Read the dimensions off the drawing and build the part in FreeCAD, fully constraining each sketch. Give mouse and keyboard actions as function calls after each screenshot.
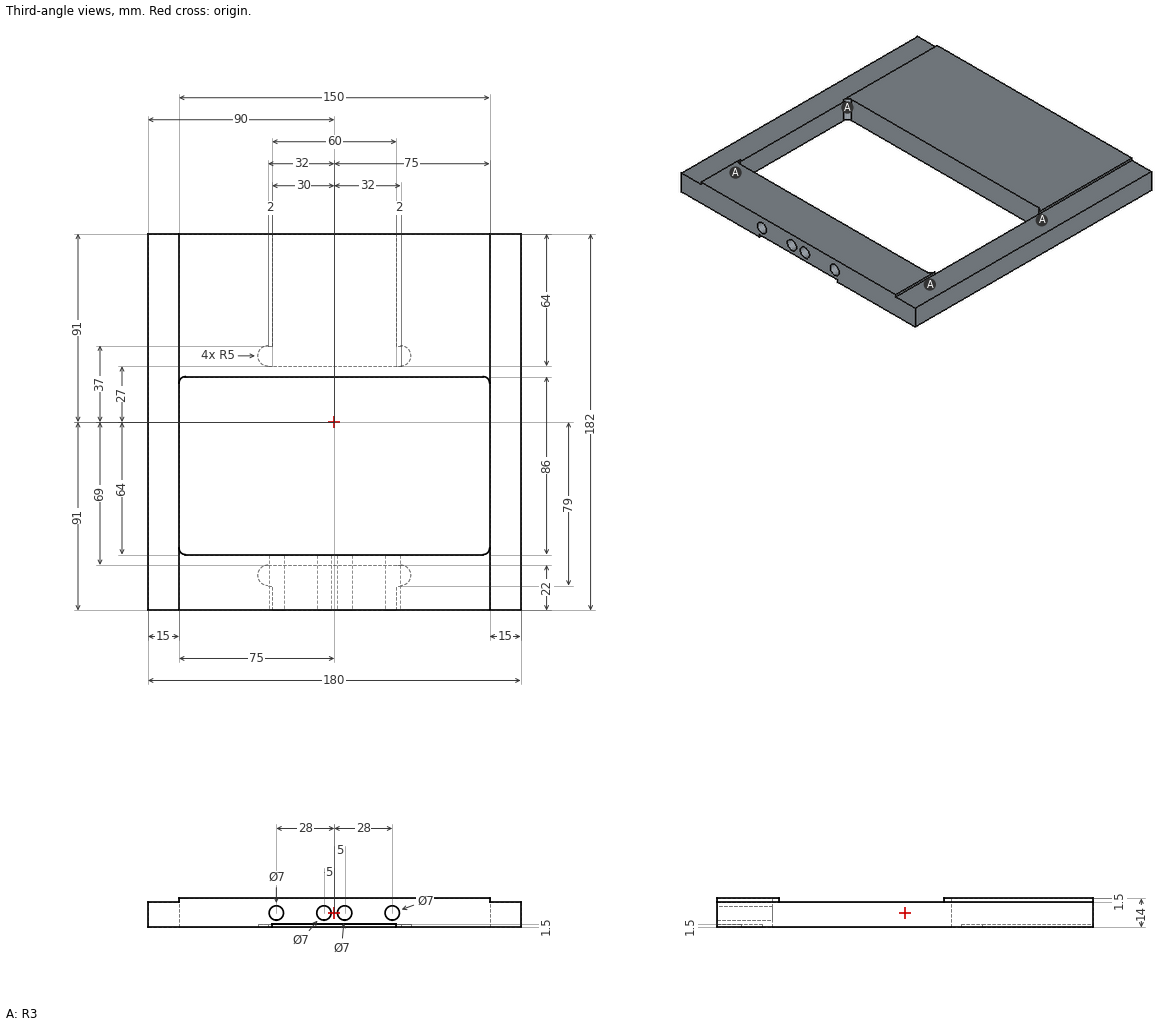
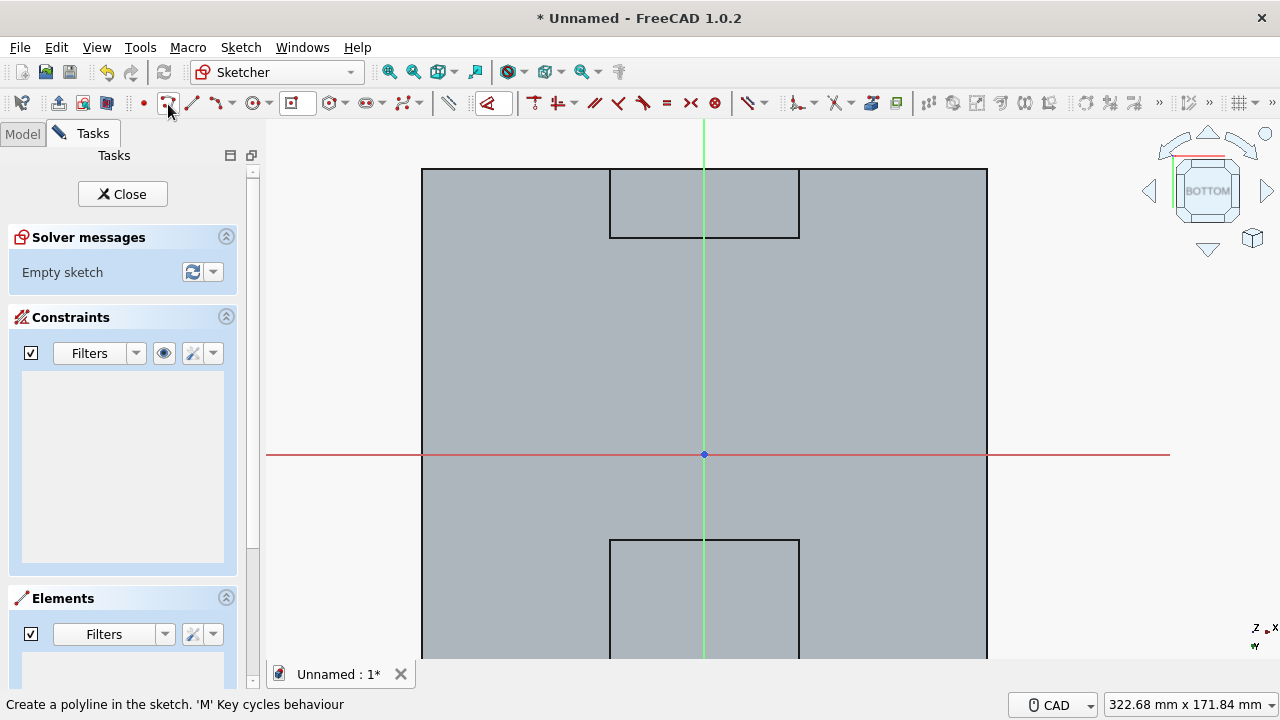
click(604, 571)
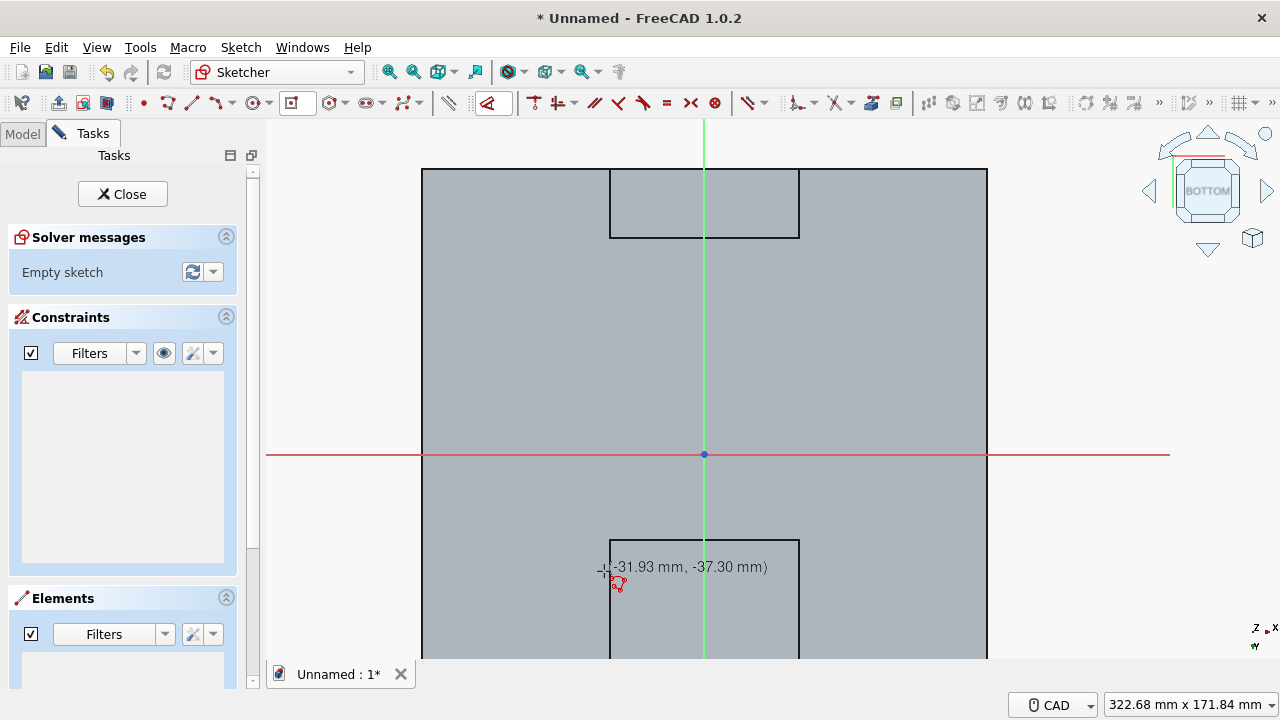
scroll(610, 571, up, 5)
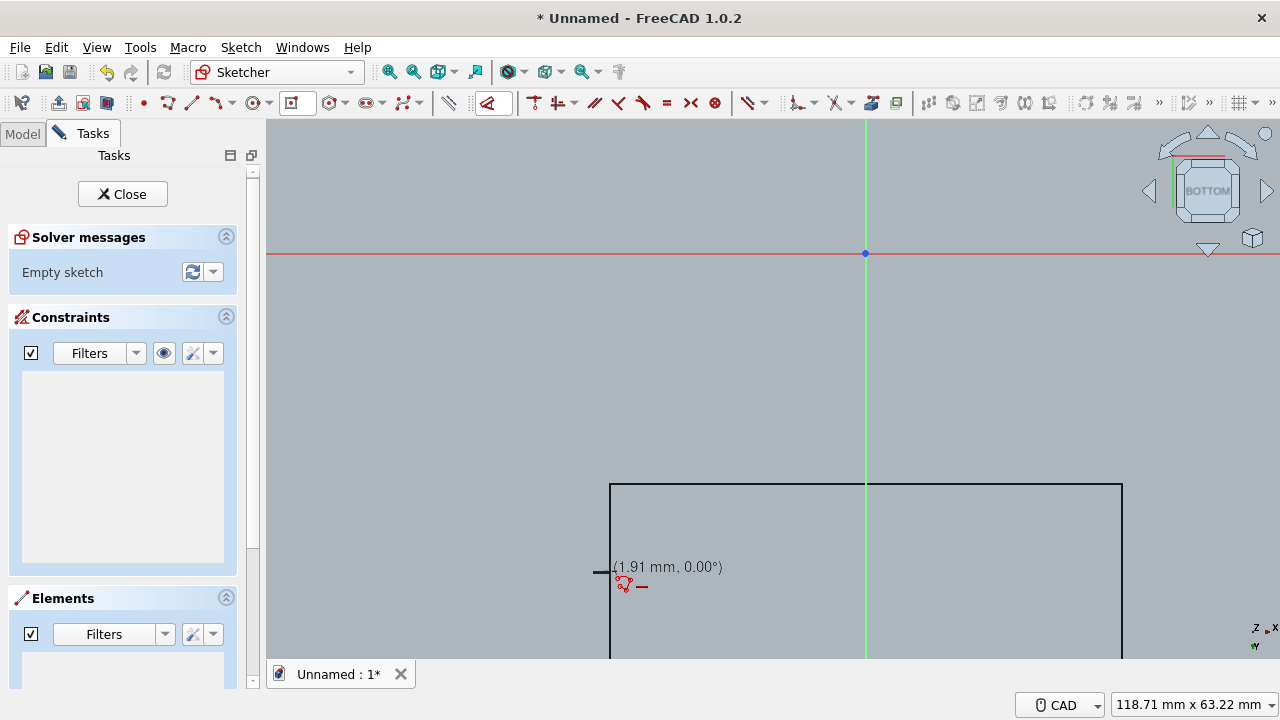
click(610, 570)
click(610, 484)
click(592, 484)
right_click(592, 484)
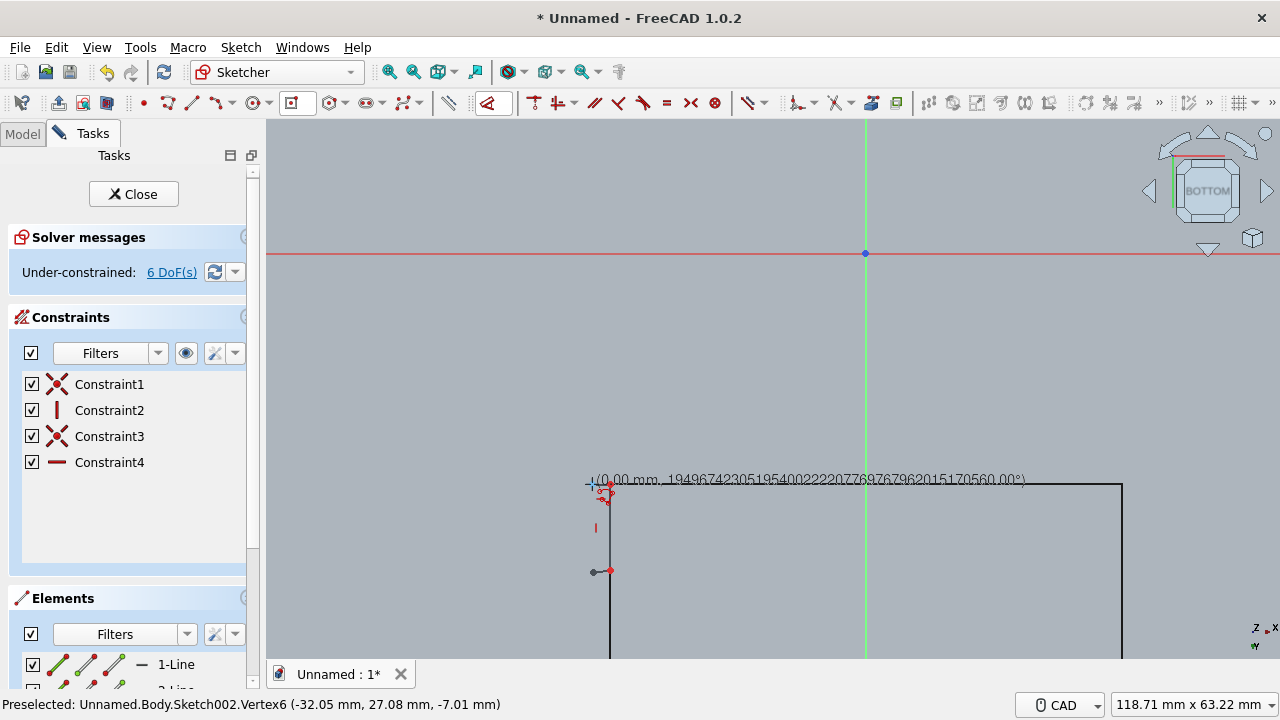
key(g)
key(3)
key(a)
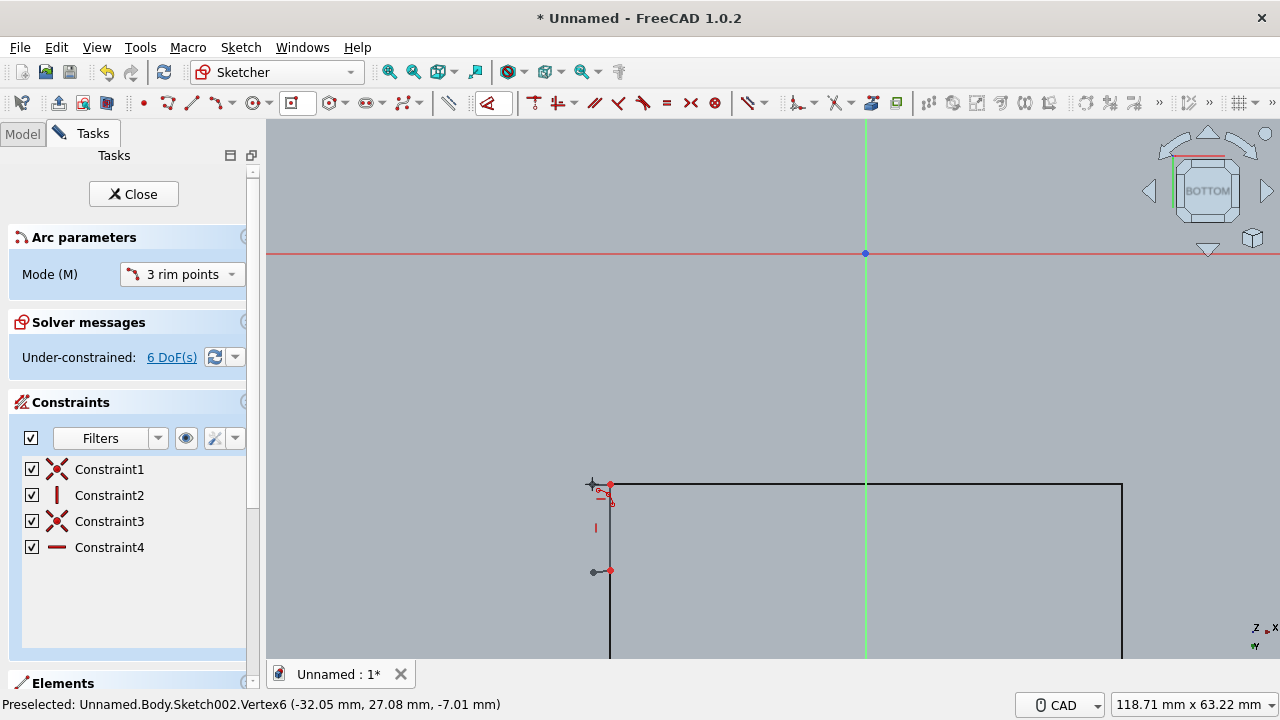
scroll(592, 484, up, 4)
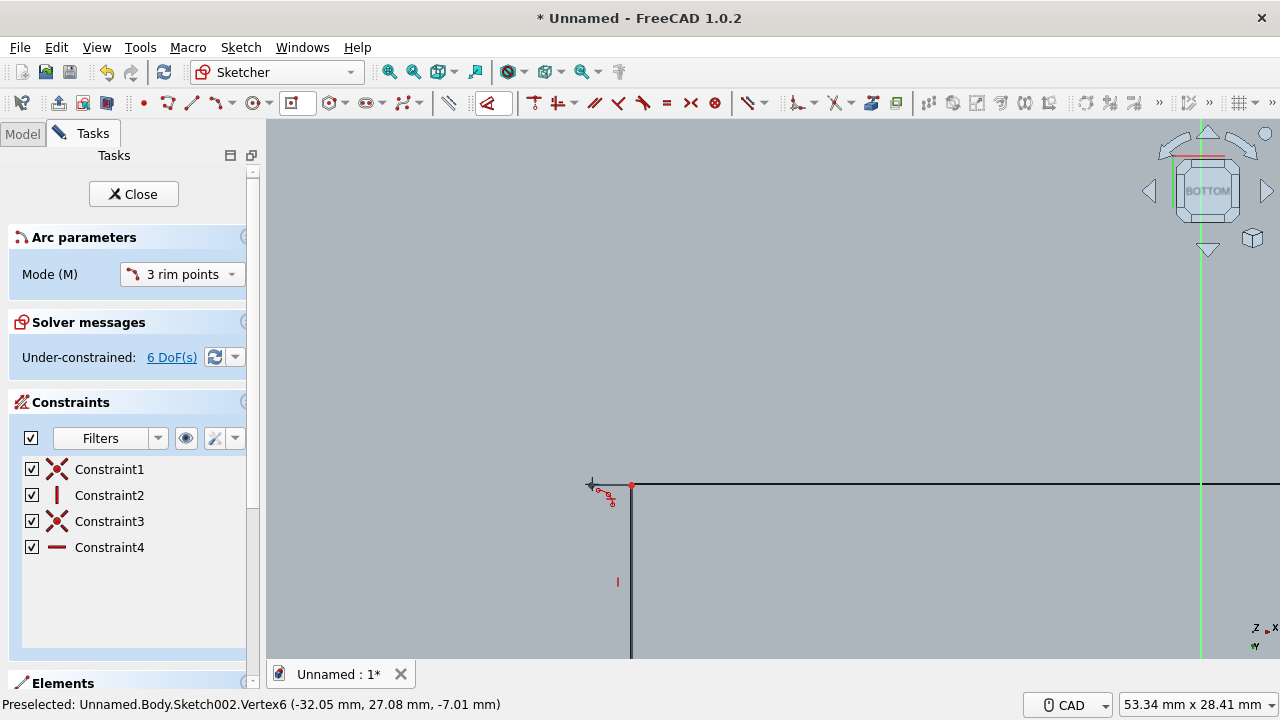
click(592, 485)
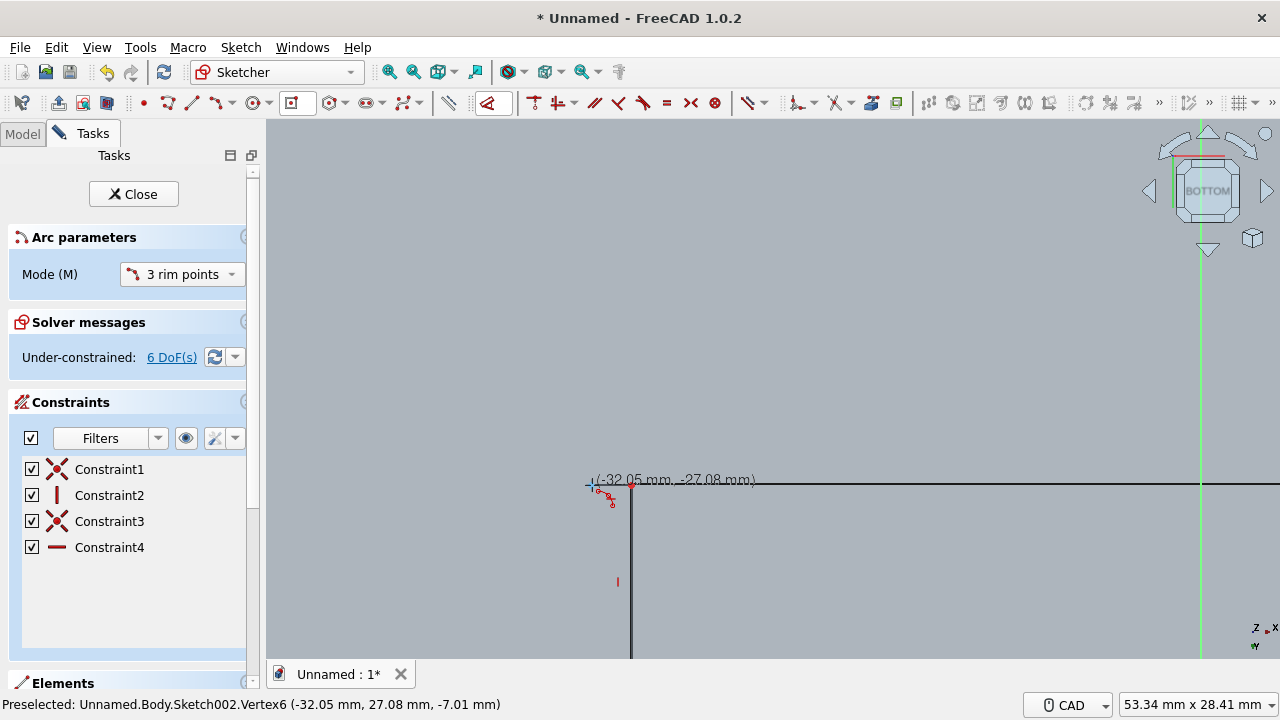
scroll(606, 551, down, 9)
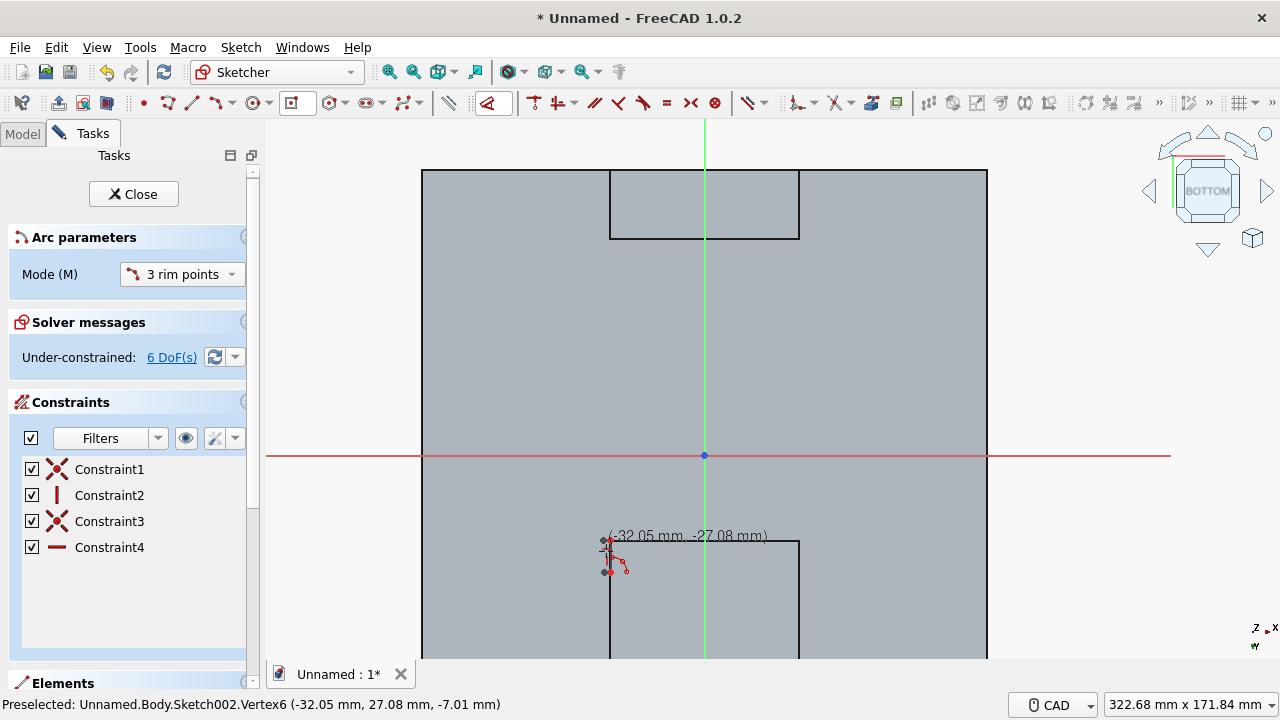
scroll(604, 572, up, 9)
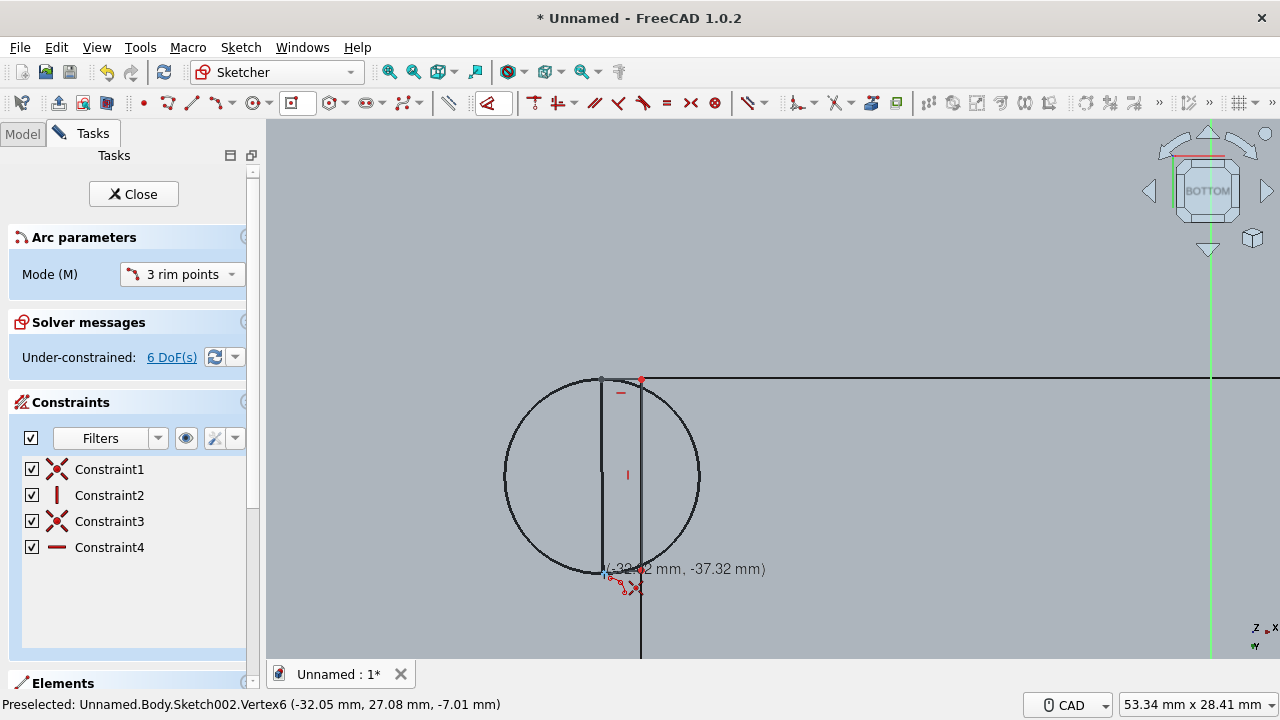
click(604, 573)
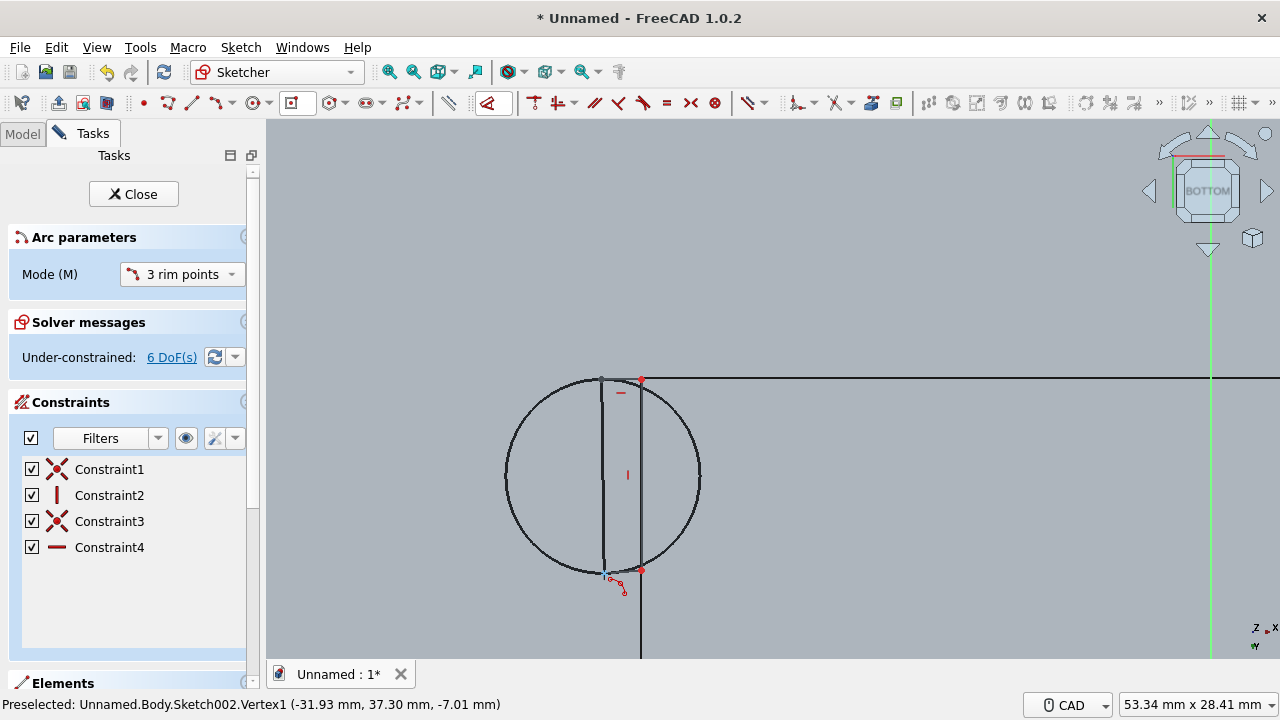
scroll(604, 572, down, 9)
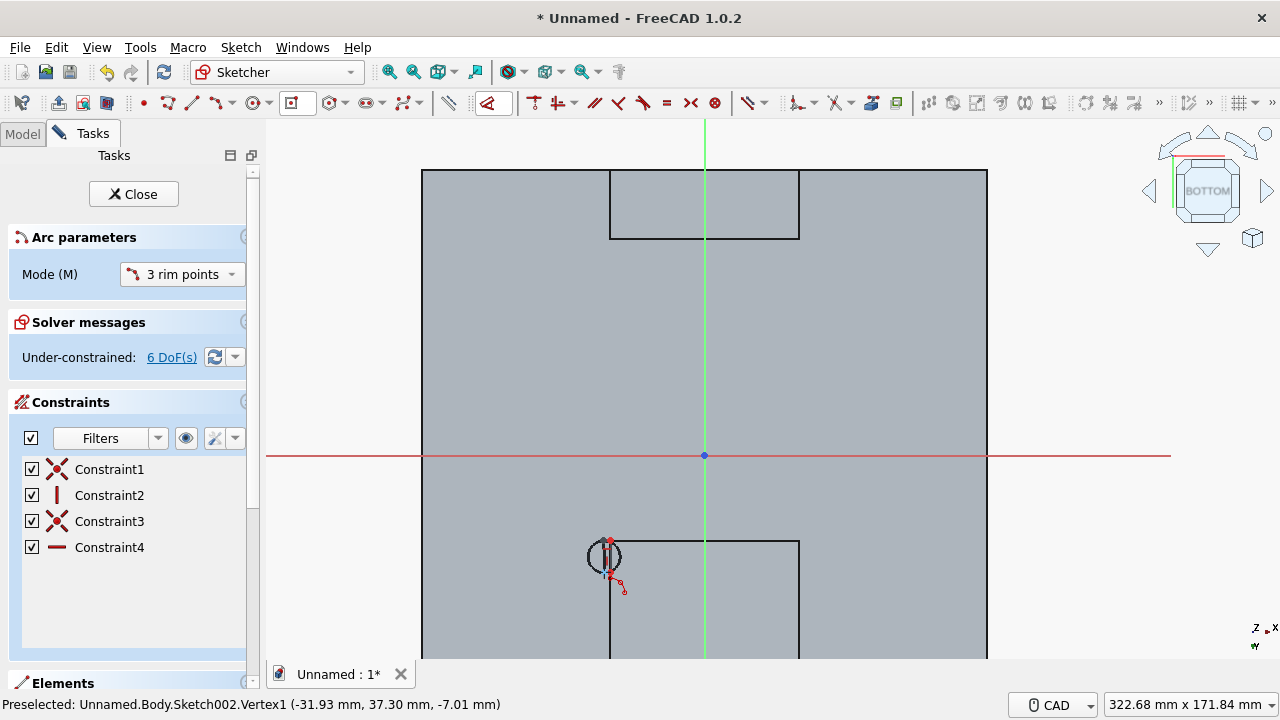
click(588, 556)